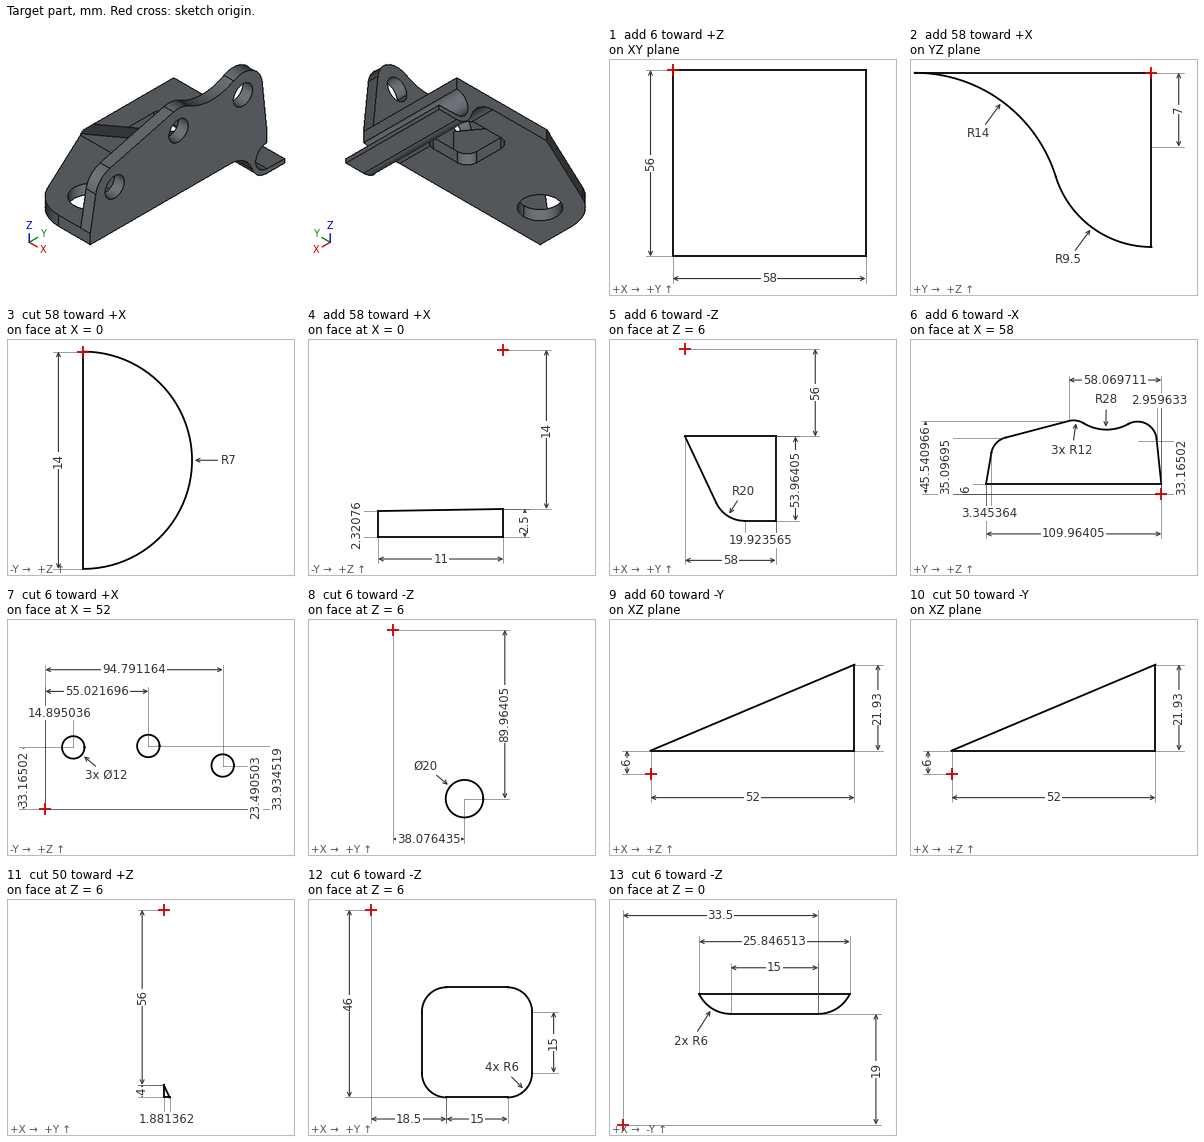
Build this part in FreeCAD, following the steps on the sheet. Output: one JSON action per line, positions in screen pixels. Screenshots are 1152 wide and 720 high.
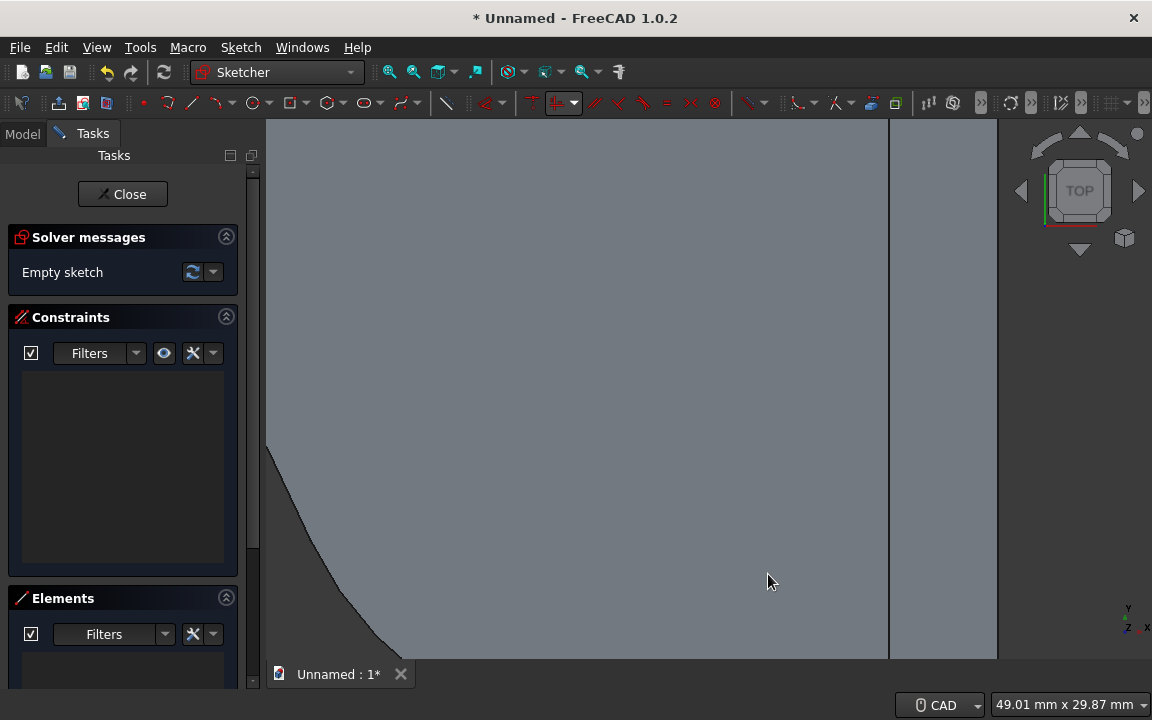
{"action": "key", "text": "g c"}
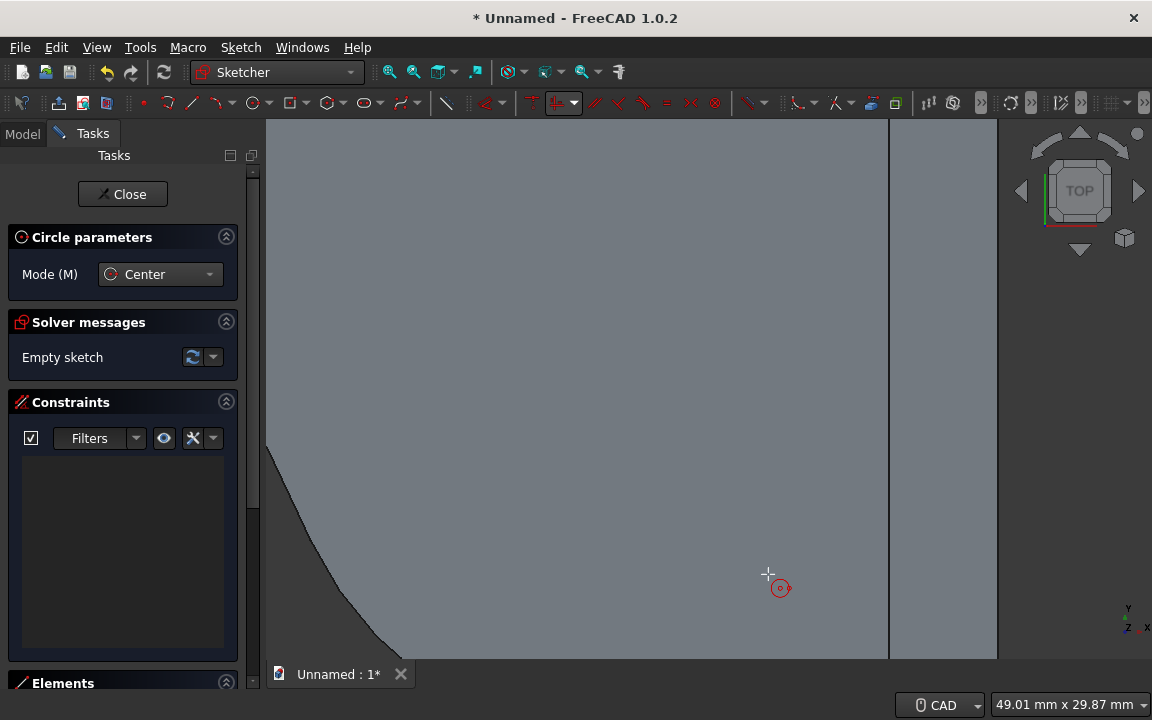
{"action": "left_click", "coordinate": [638, 386]}
{"action": "left_click", "coordinate": [765, 258]}
{"action": "key", "text": "Escape"}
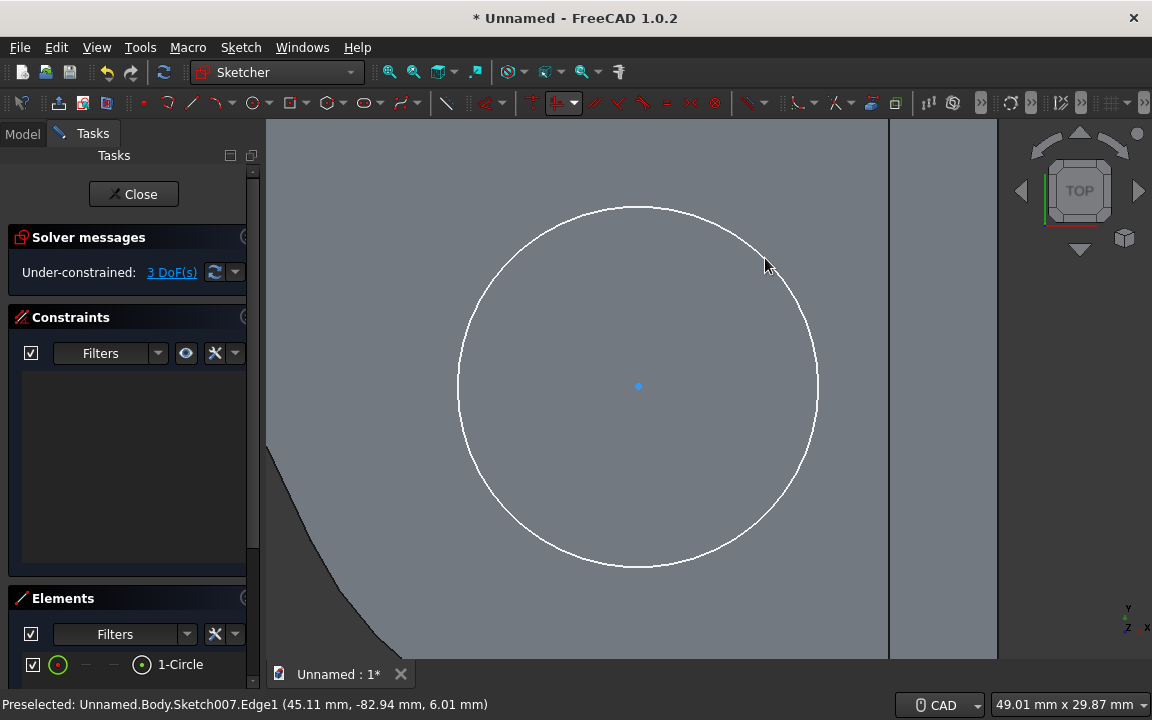
{"action": "left_click", "coordinate": [486, 104]}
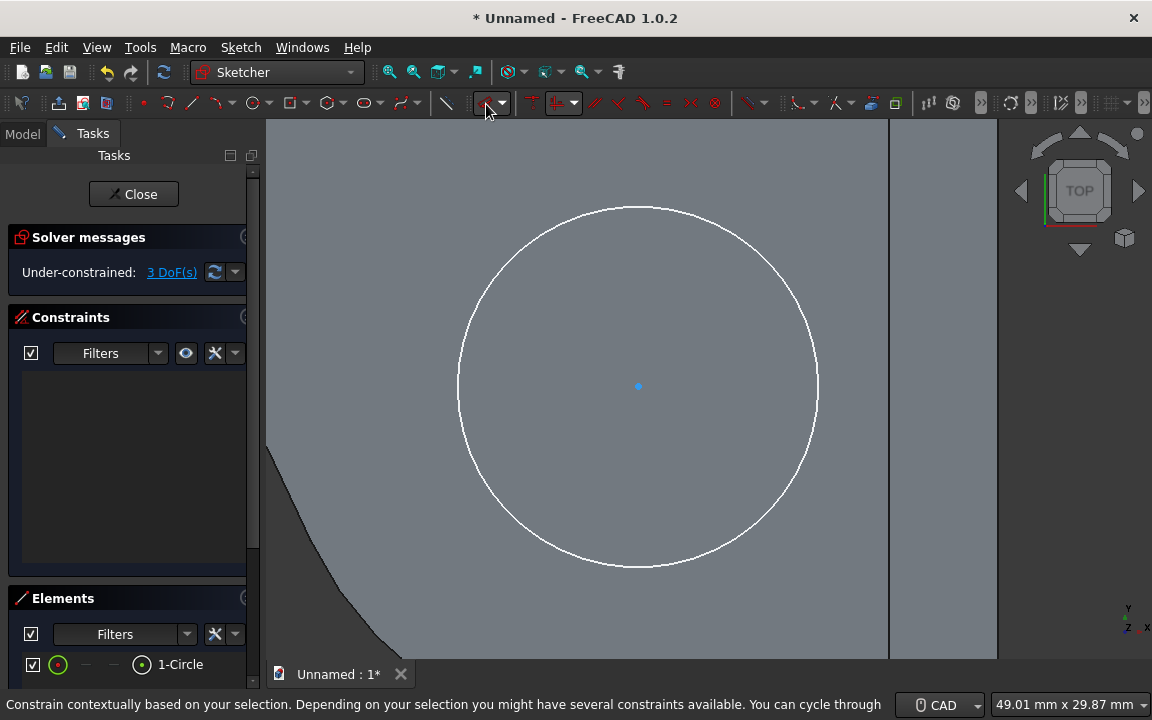
{"action": "left_click", "coordinate": [765, 259]}
{"action": "left_click", "coordinate": [788, 236]}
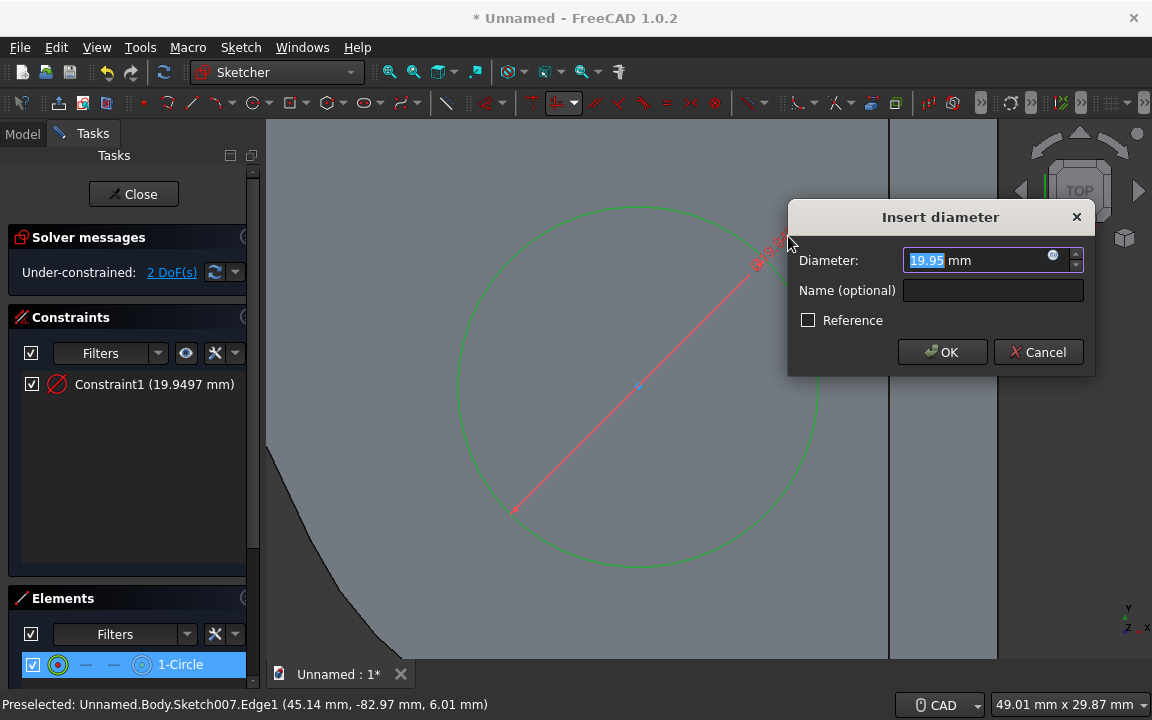
{"action": "type", "text": "20"}
{"action": "key", "text": "Return"}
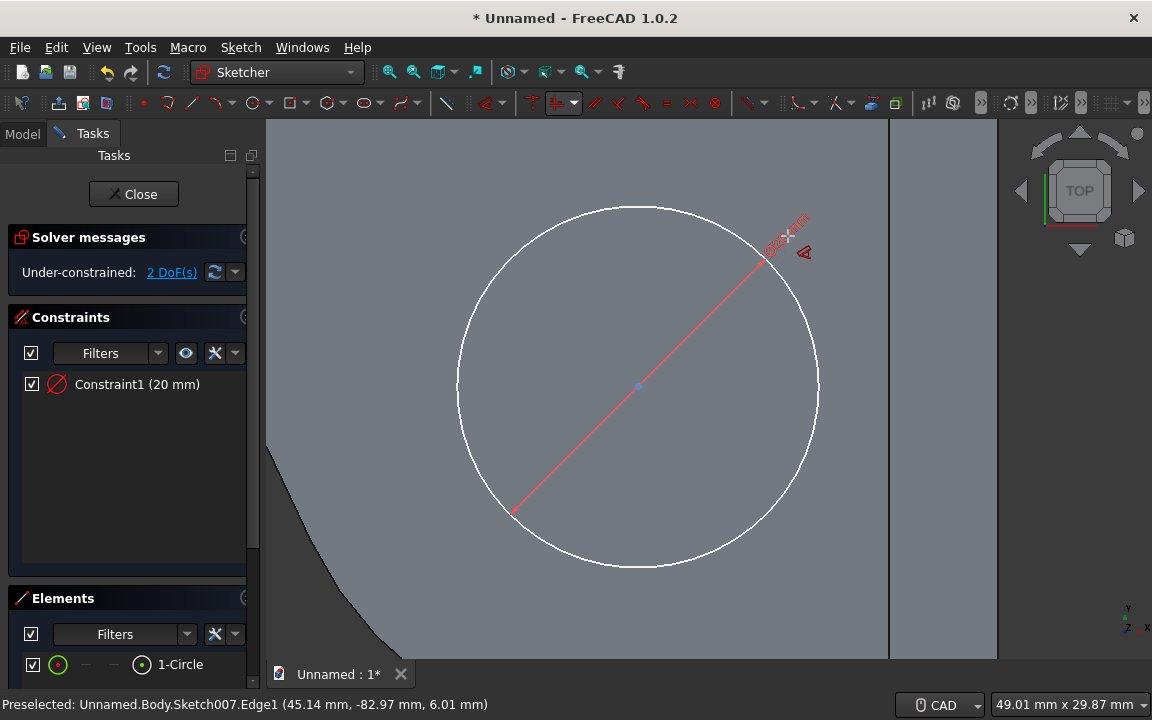
{"action": "left_click", "coordinate": [638, 387]}
{"action": "left_click", "coordinate": [672, 267]}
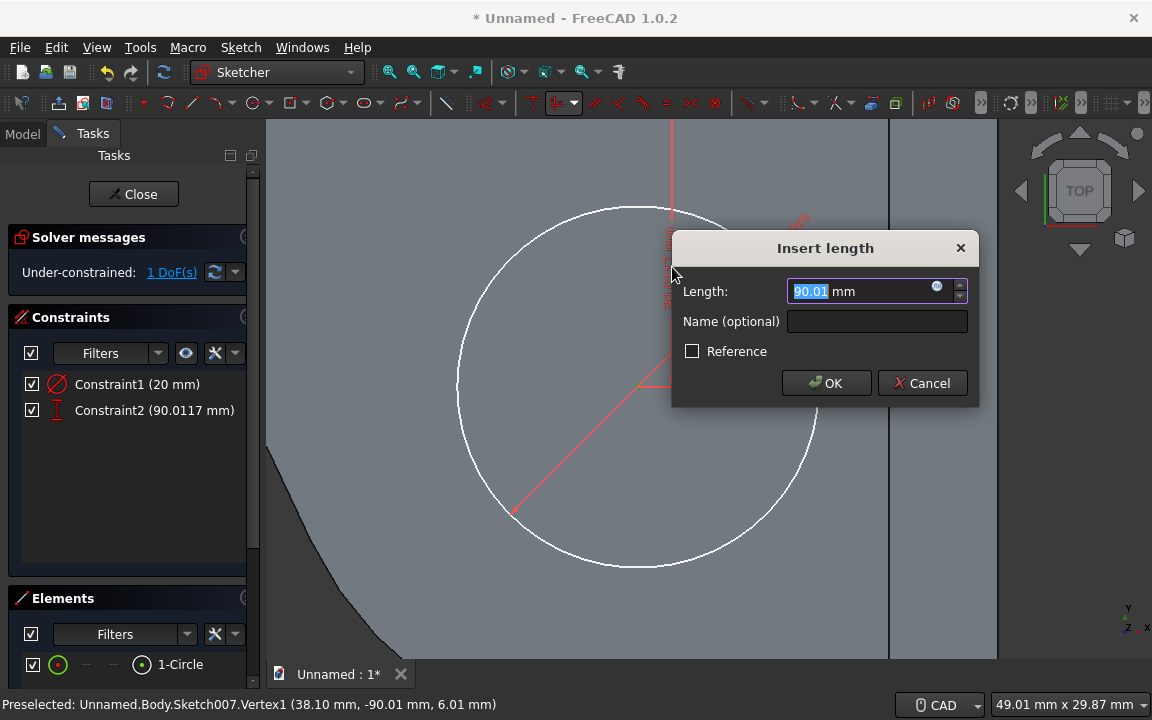
{"action": "type", "text": "89.96405"}
{"action": "key", "text": "Return"}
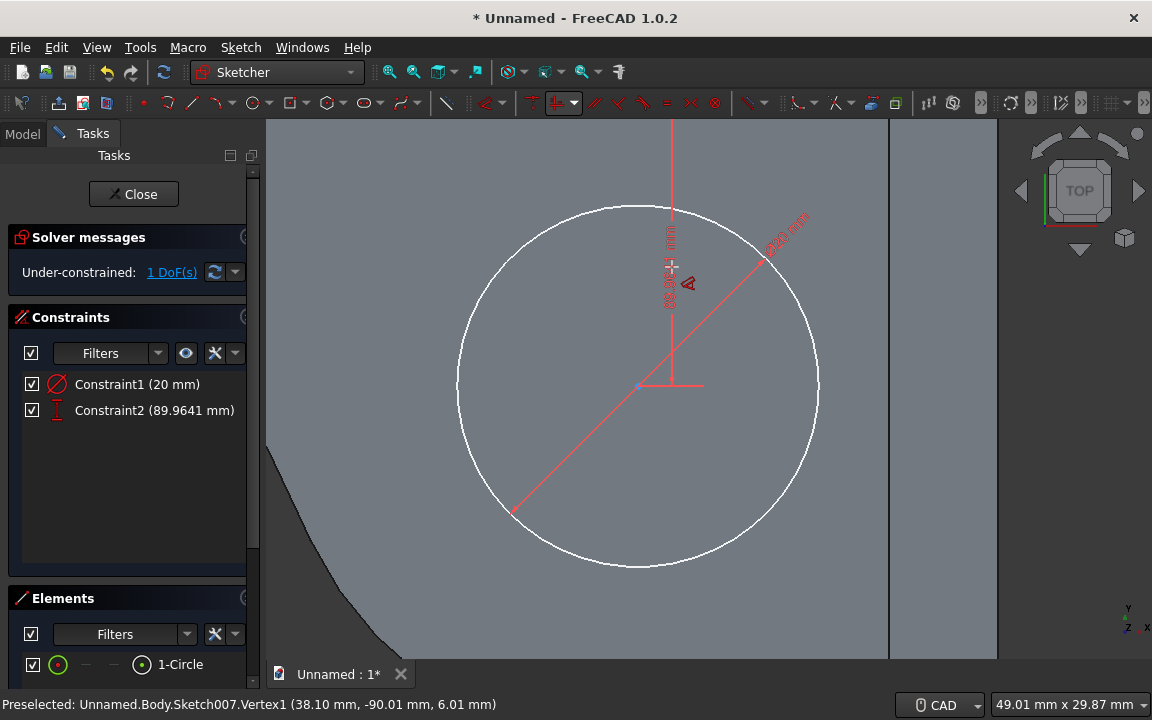
{"action": "left_click", "coordinate": [638, 386]}
{"action": "left_click", "coordinate": [387, 420]}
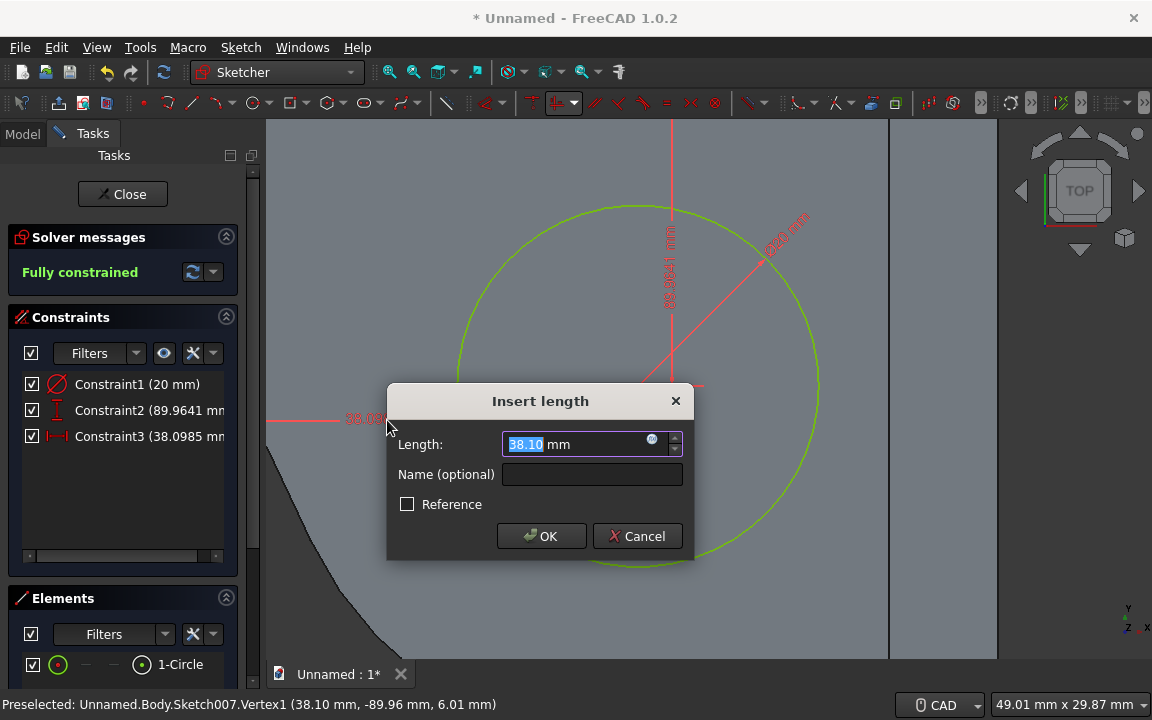
{"action": "type", "text": "38.076435"}
{"action": "key", "text": "Return"}
{"action": "key", "text": "Escape"}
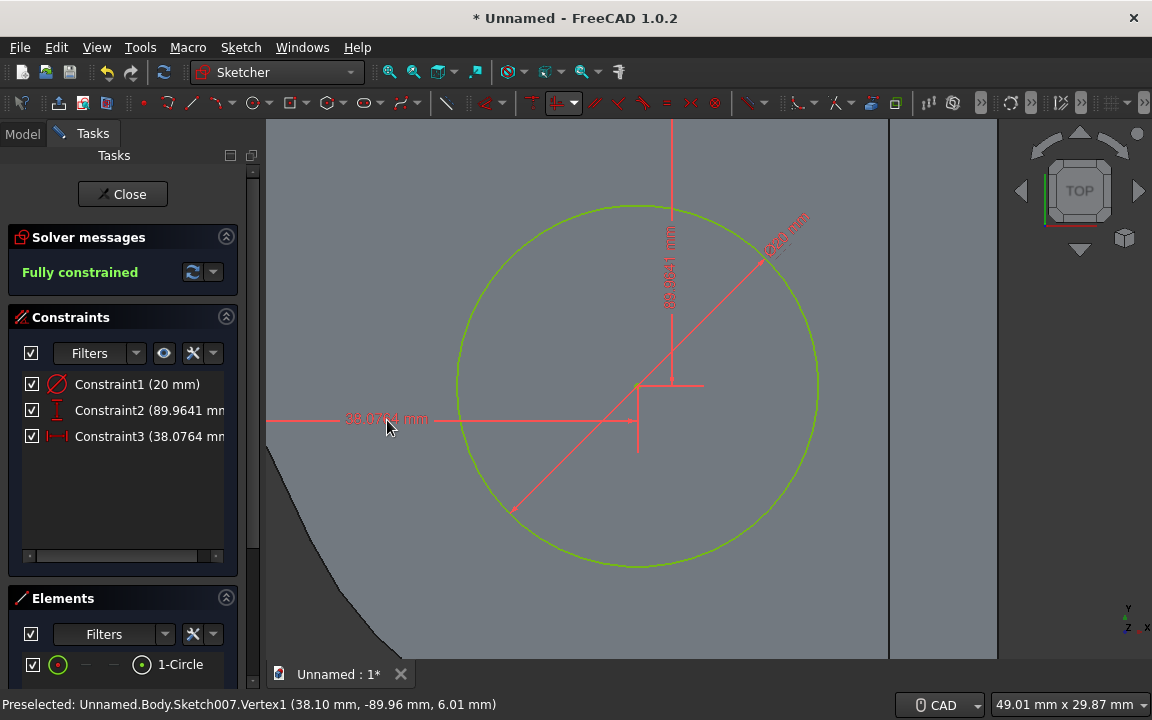
{"action": "left_click", "coordinate": [123, 194]}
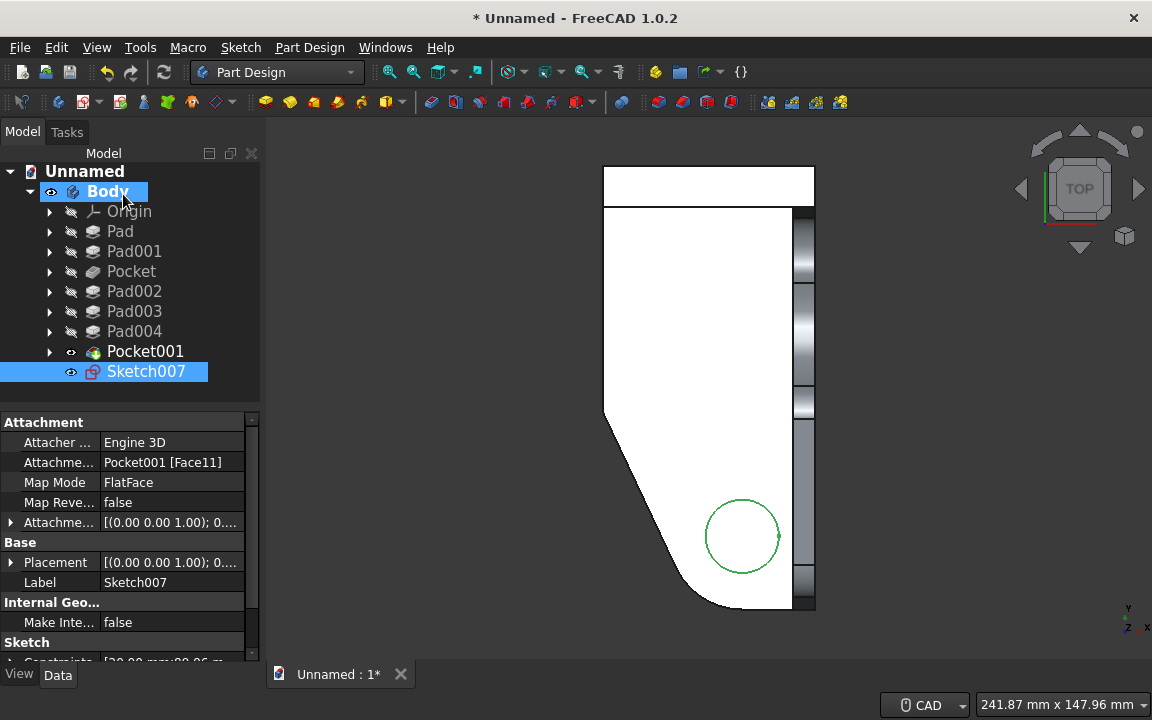
{"action": "left_click", "coordinate": [432, 102]}